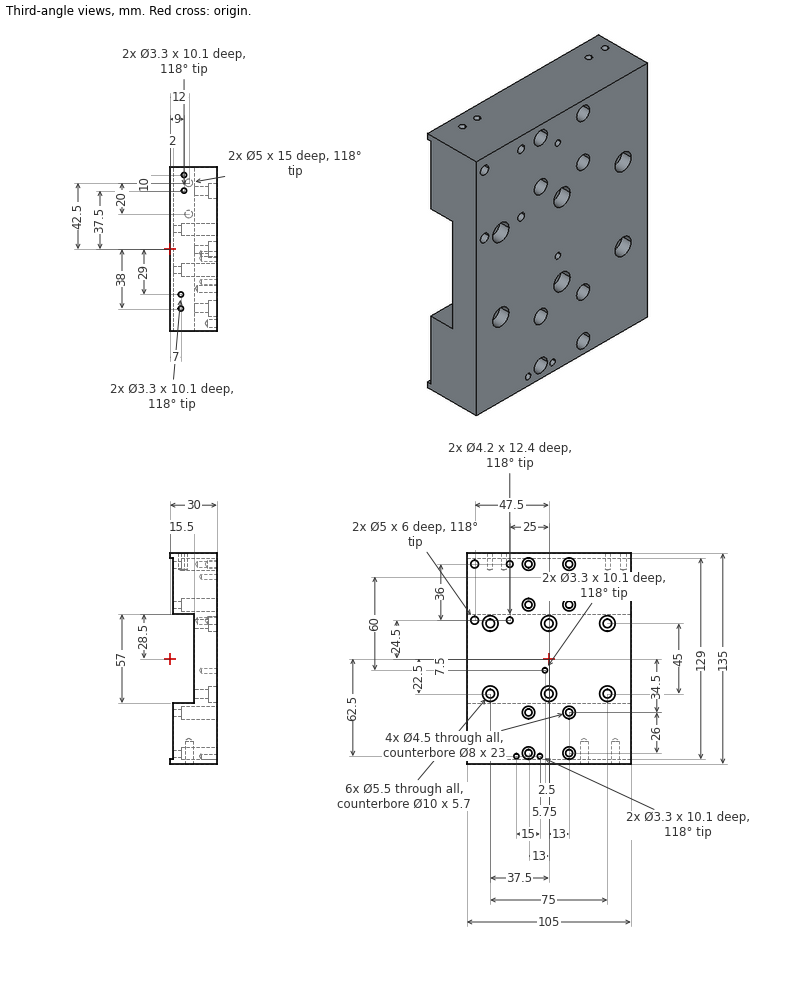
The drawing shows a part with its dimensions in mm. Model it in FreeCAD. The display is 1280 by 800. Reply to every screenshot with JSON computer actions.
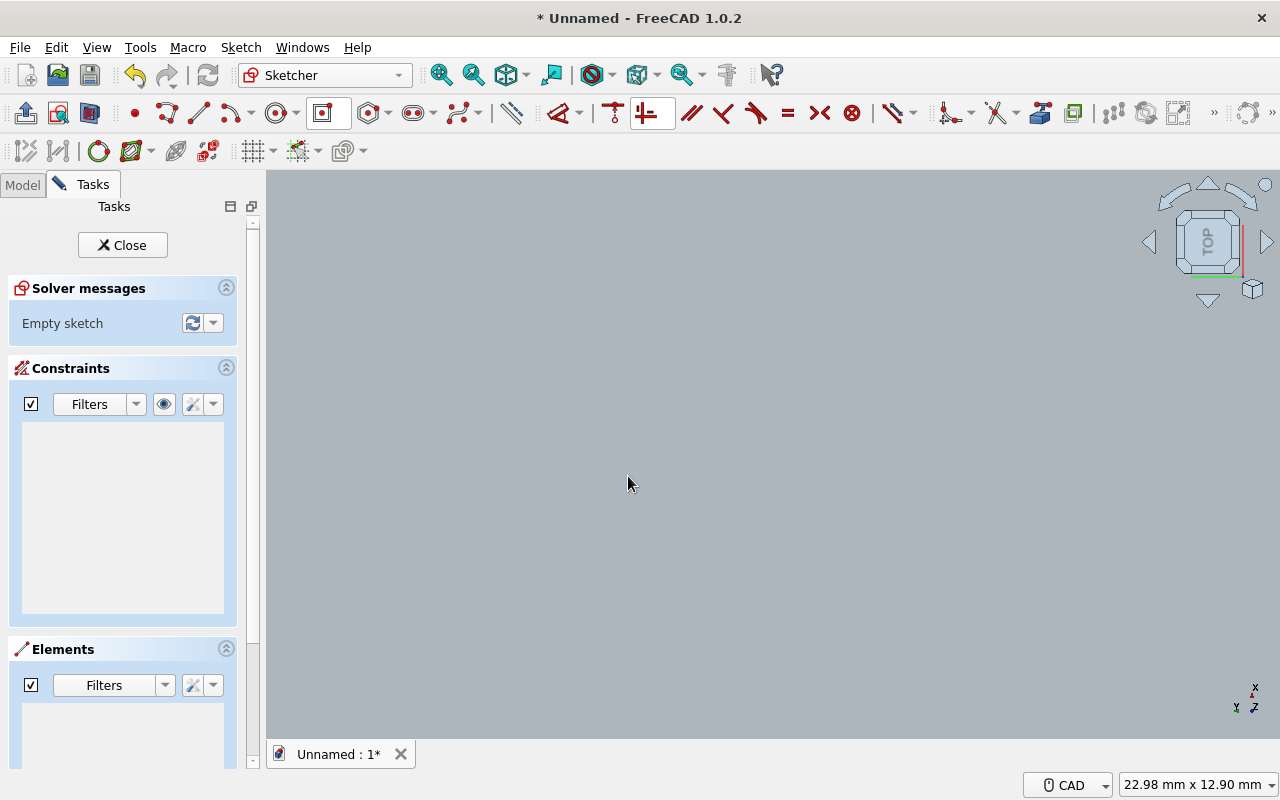
{"action": "left_click", "coordinate": [276, 114]}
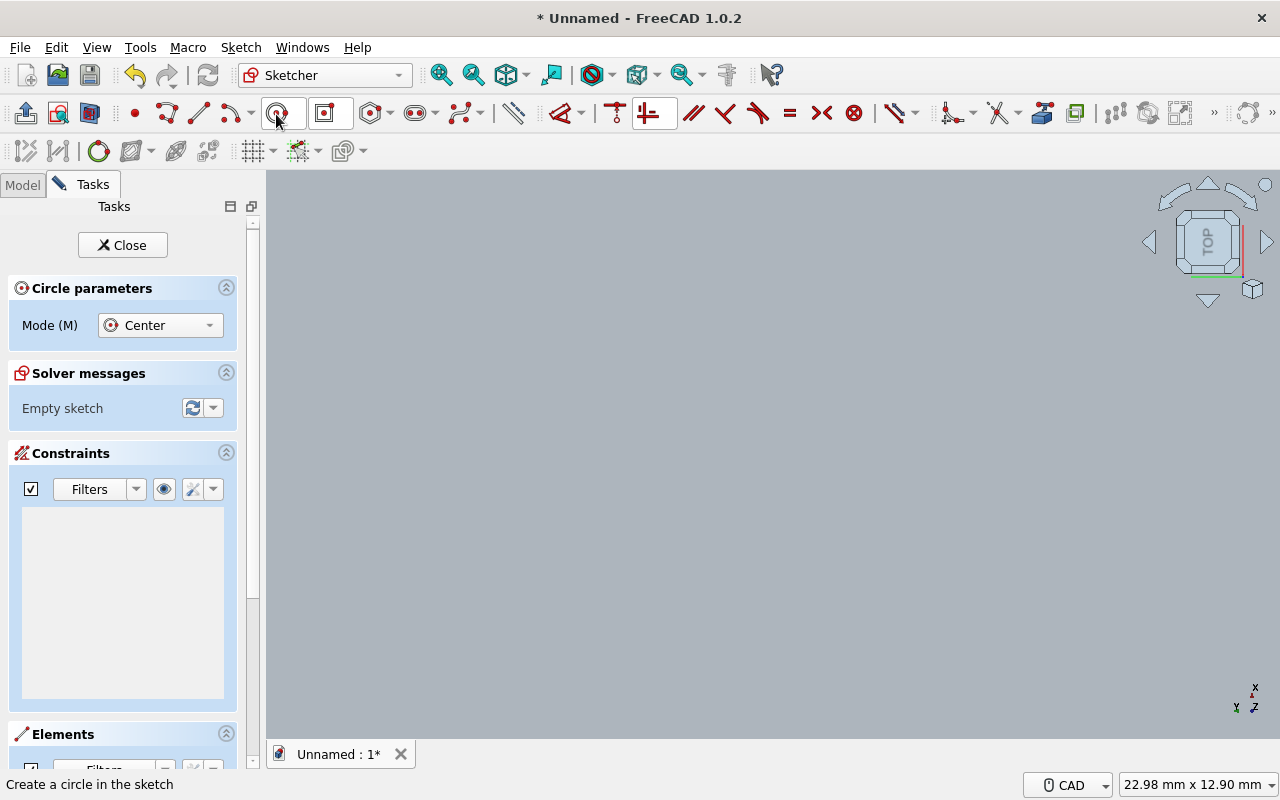
{"action": "left_click", "coordinate": [921, 445]}
{"action": "left_click", "coordinate": [973, 393]}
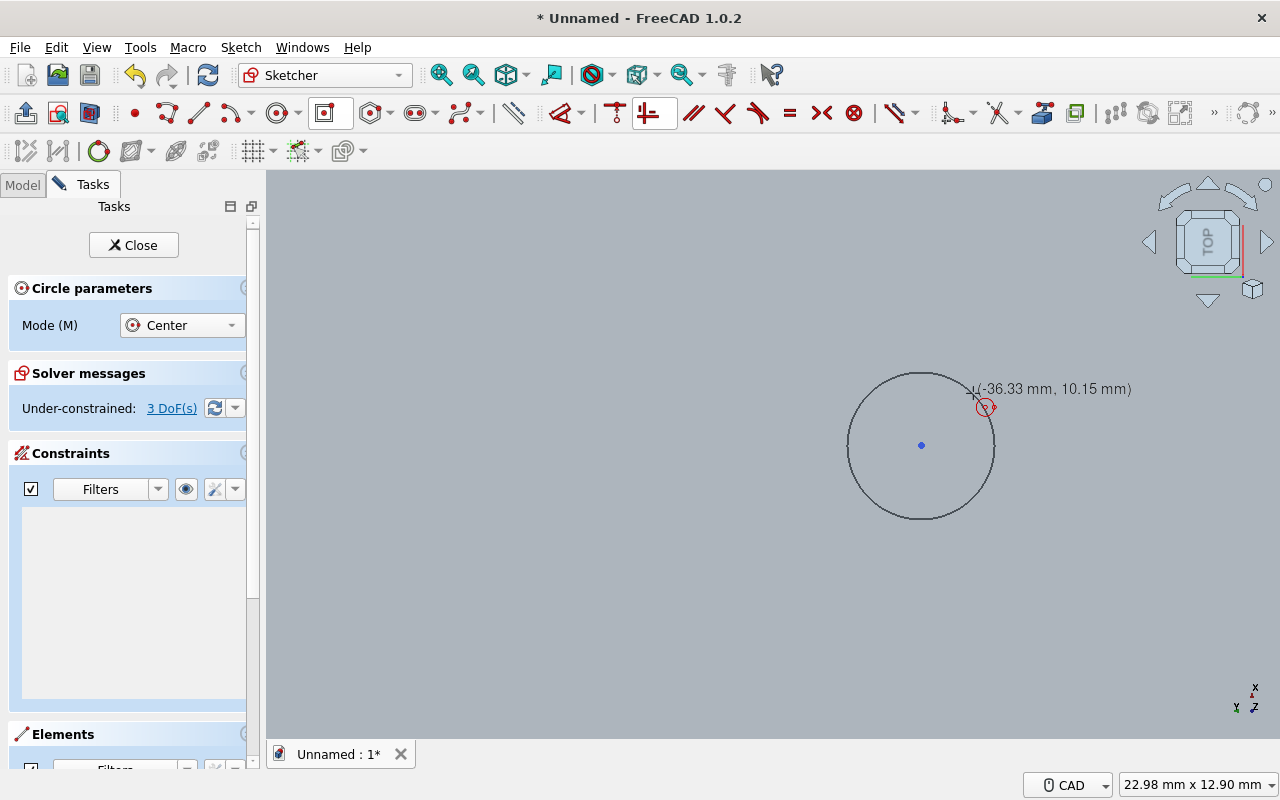
{"action": "left_click", "coordinate": [480, 445]}
{"action": "left_click", "coordinate": [532, 393]}
{"action": "key", "text": "Escape"}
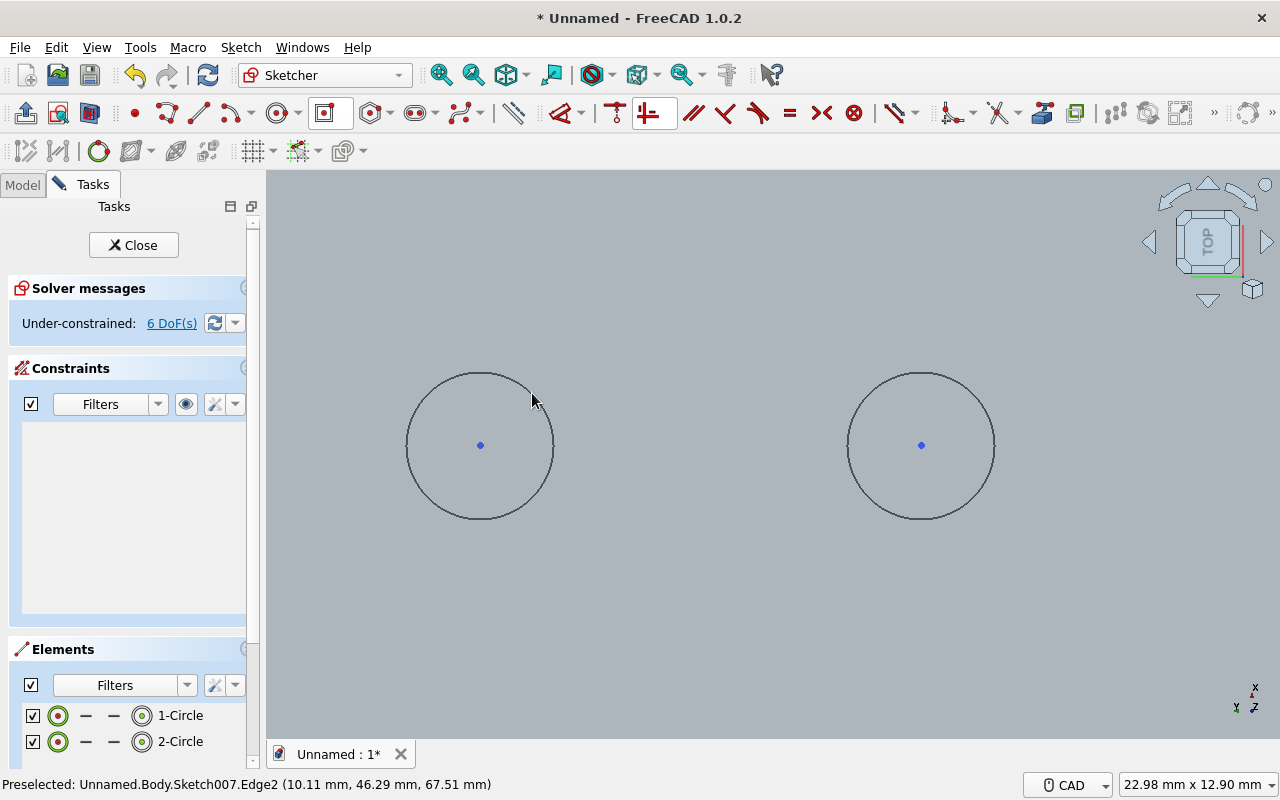
{"action": "left_click", "coordinate": [973, 394]}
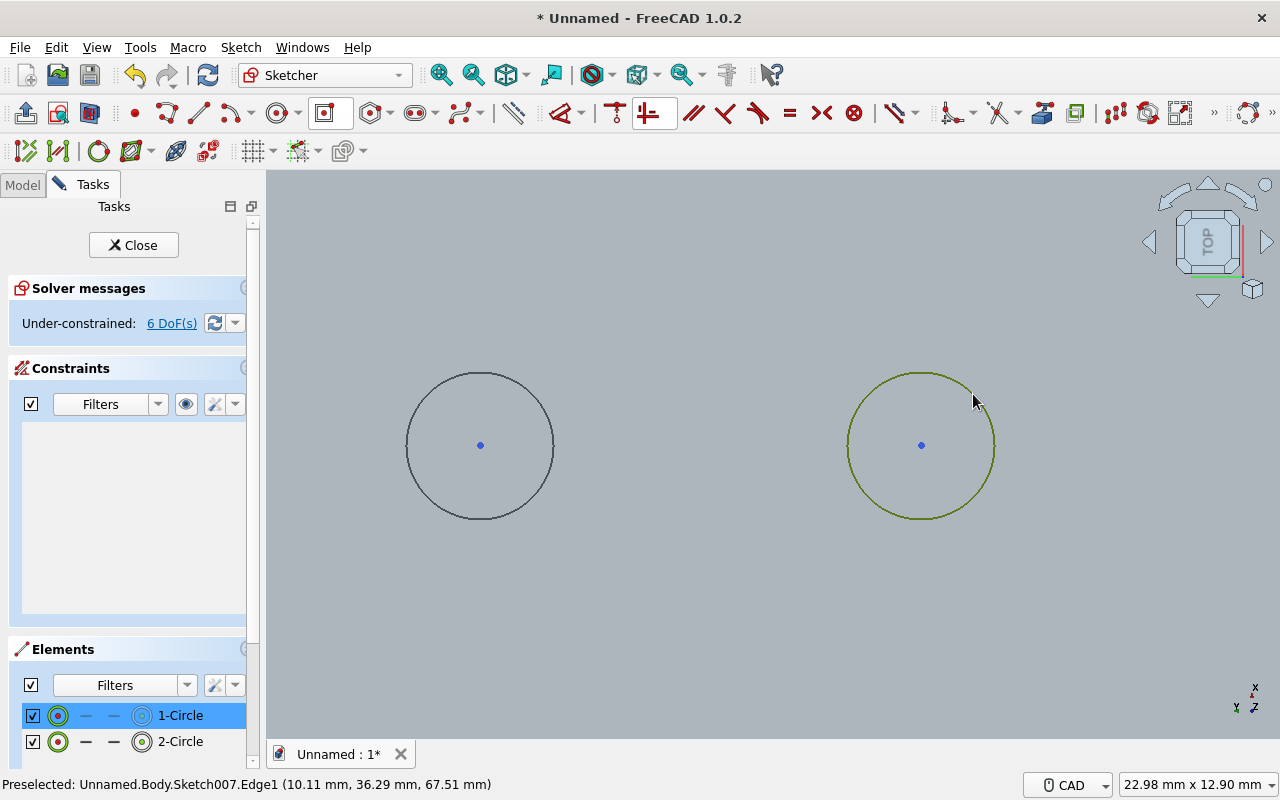
{"action": "left_click", "coordinate": [532, 394]}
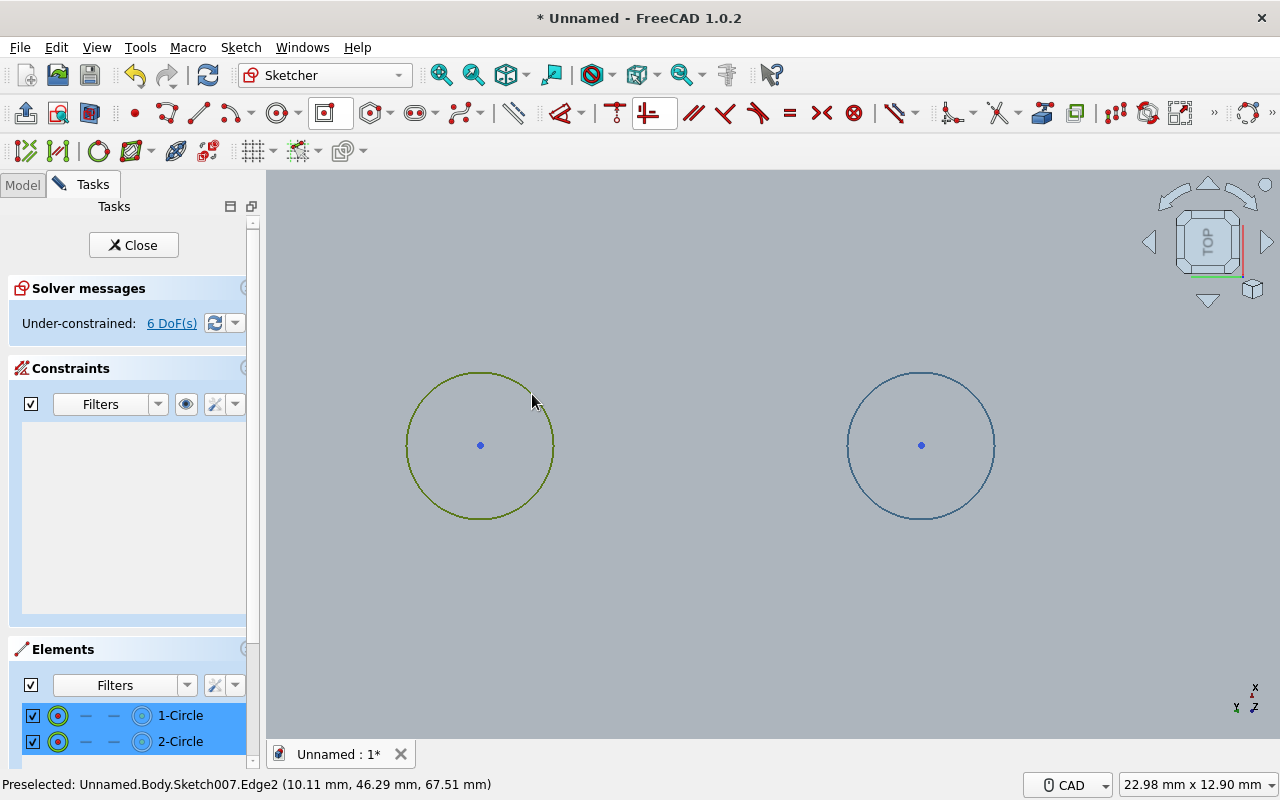
{"action": "left_click", "coordinate": [790, 114]}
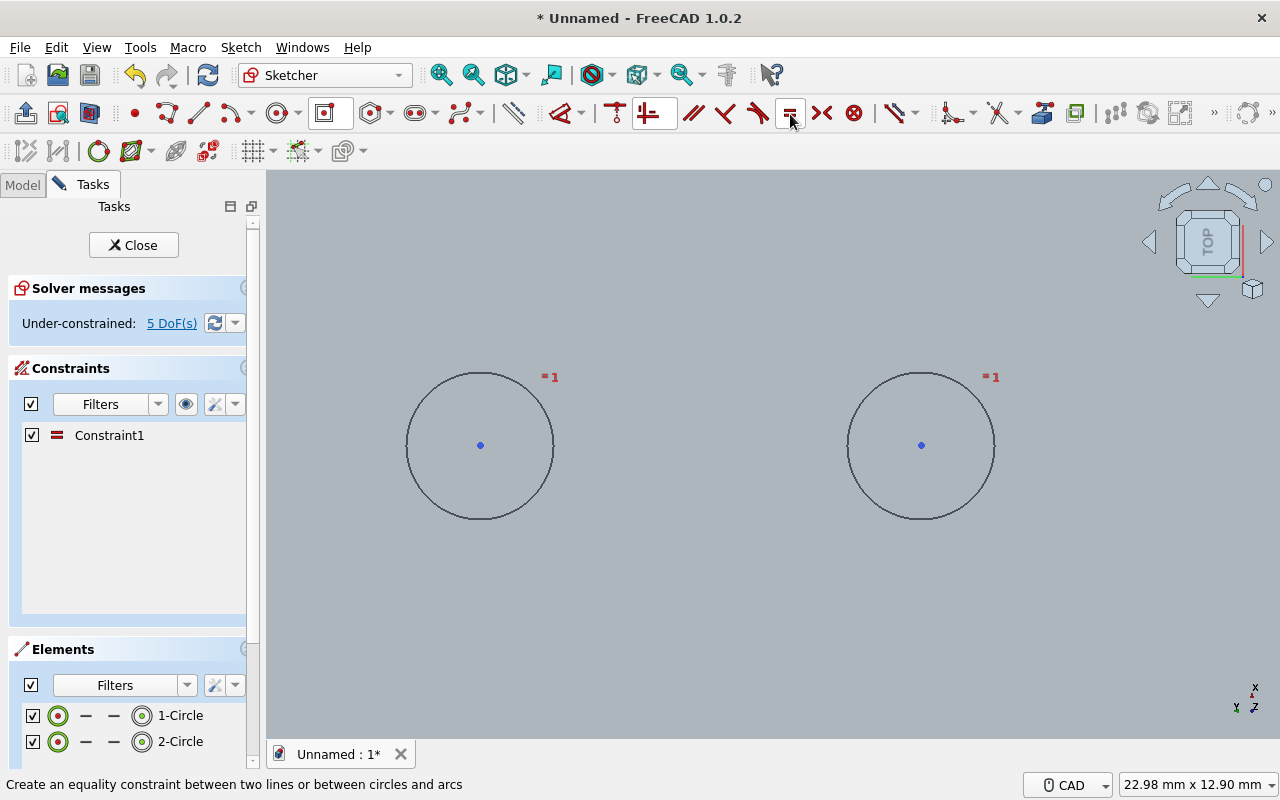
{"action": "left_click", "coordinate": [921, 446]}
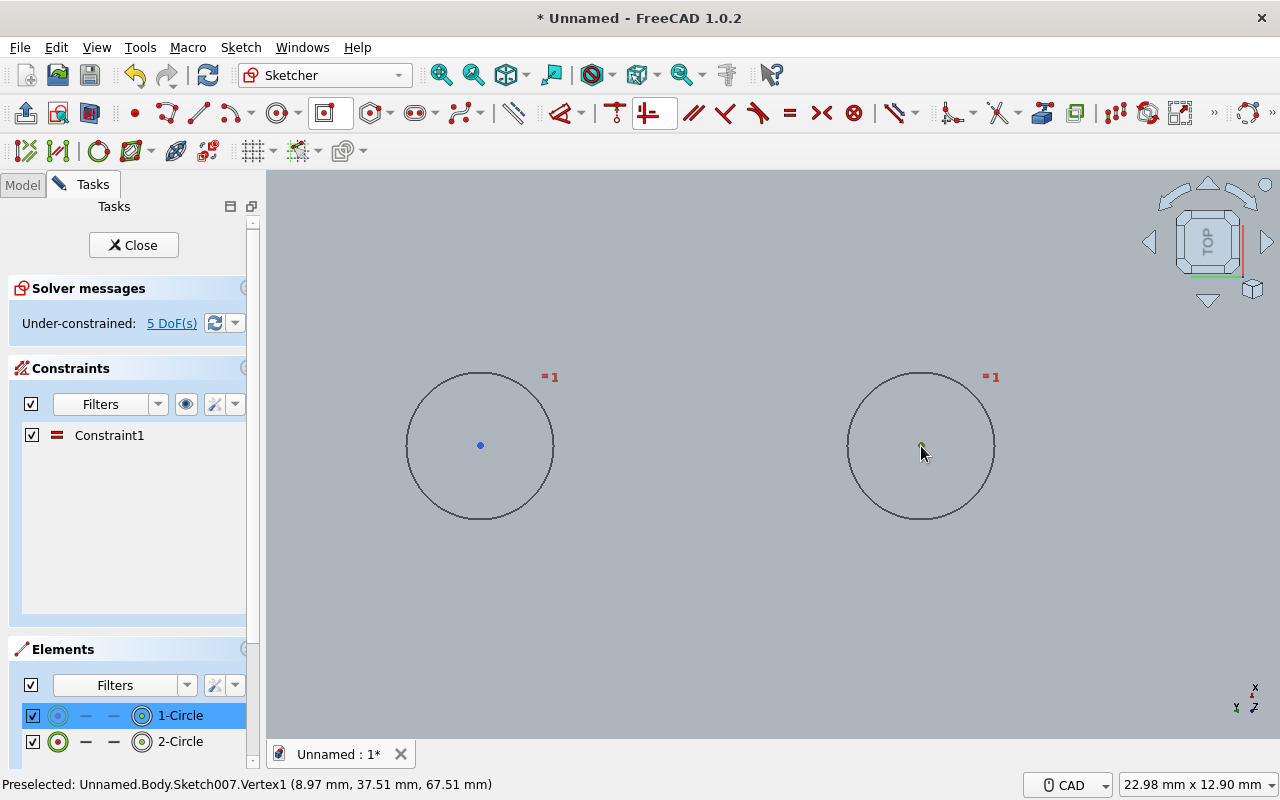
{"action": "left_click", "coordinate": [480, 446]}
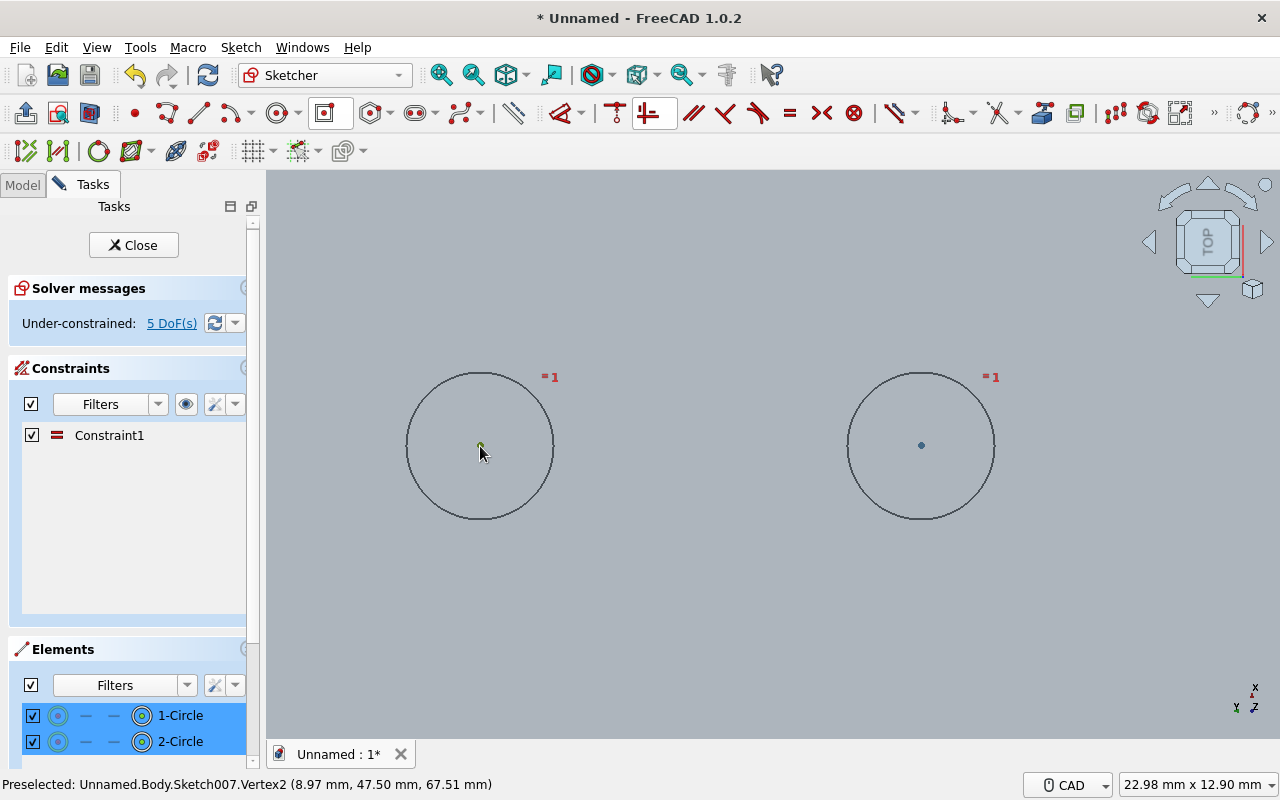
{"action": "key", "text": "h"}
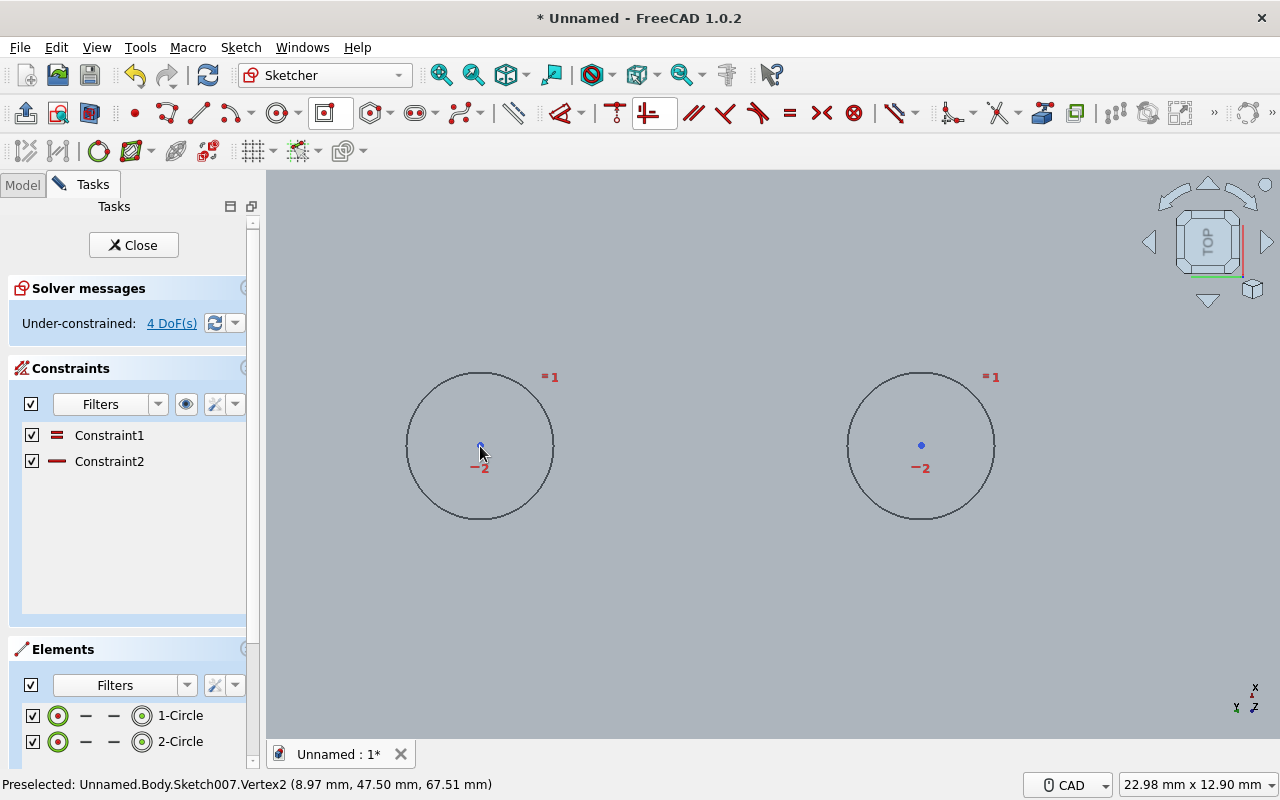
{"action": "left_click", "coordinate": [560, 114]}